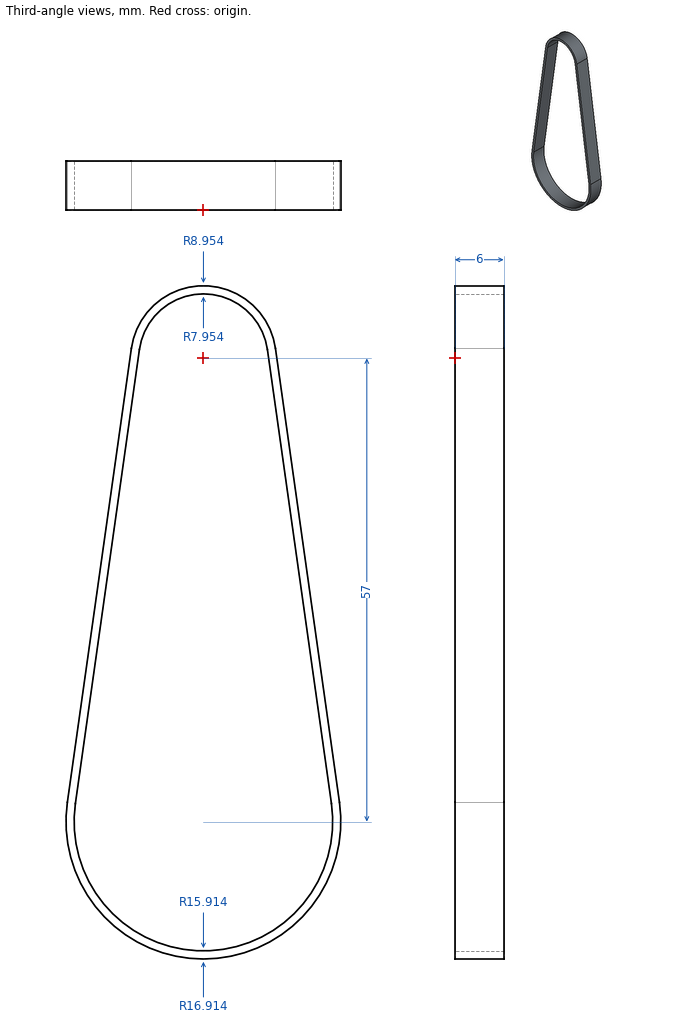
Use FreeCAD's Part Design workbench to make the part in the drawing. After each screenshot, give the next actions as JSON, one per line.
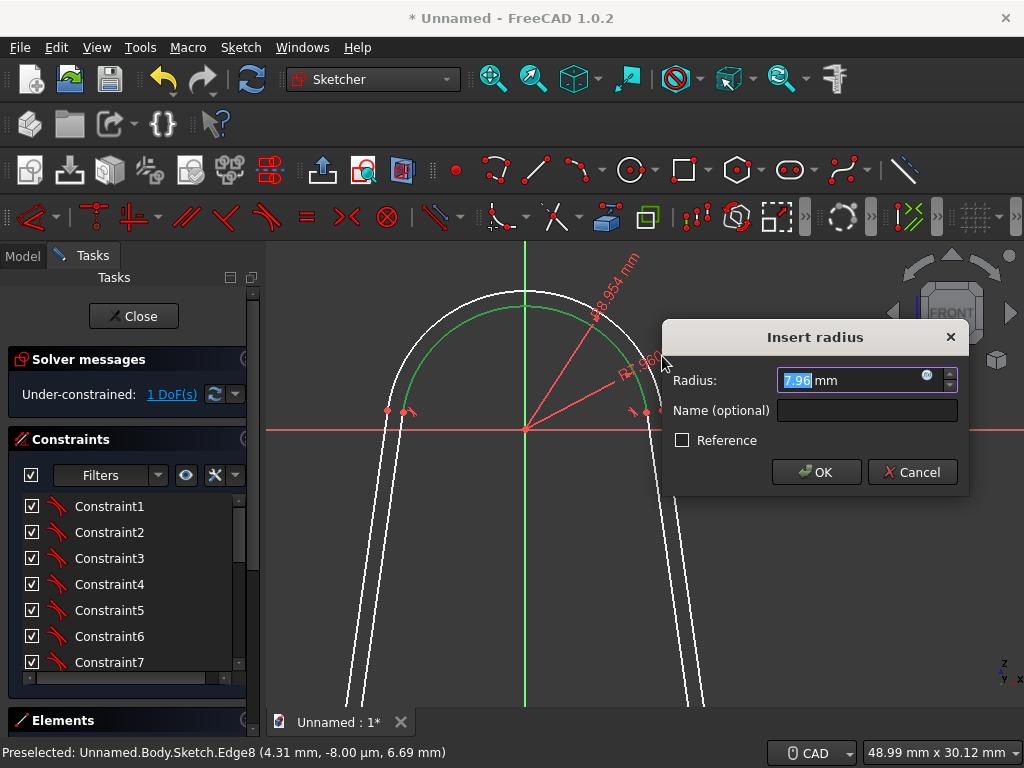
{"action": "type", "text": "7.954"}
{"action": "key", "text": "Return"}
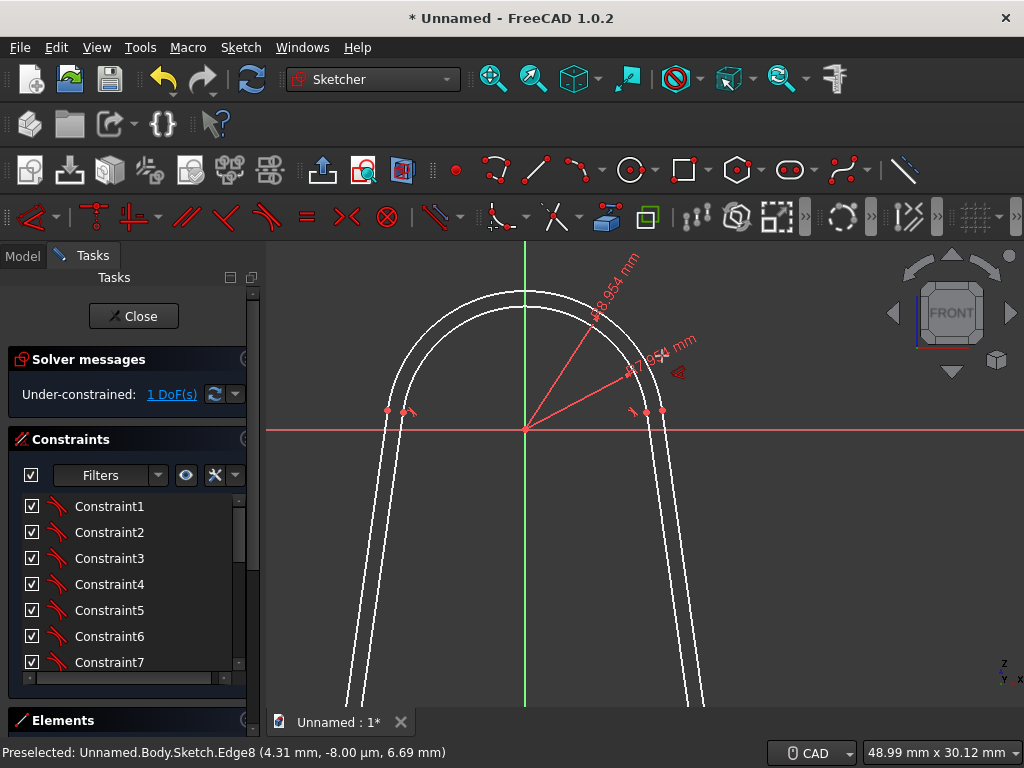
{"action": "scroll", "coordinate": [593, 324], "scroll_direction": "down", "scroll_amount": 7}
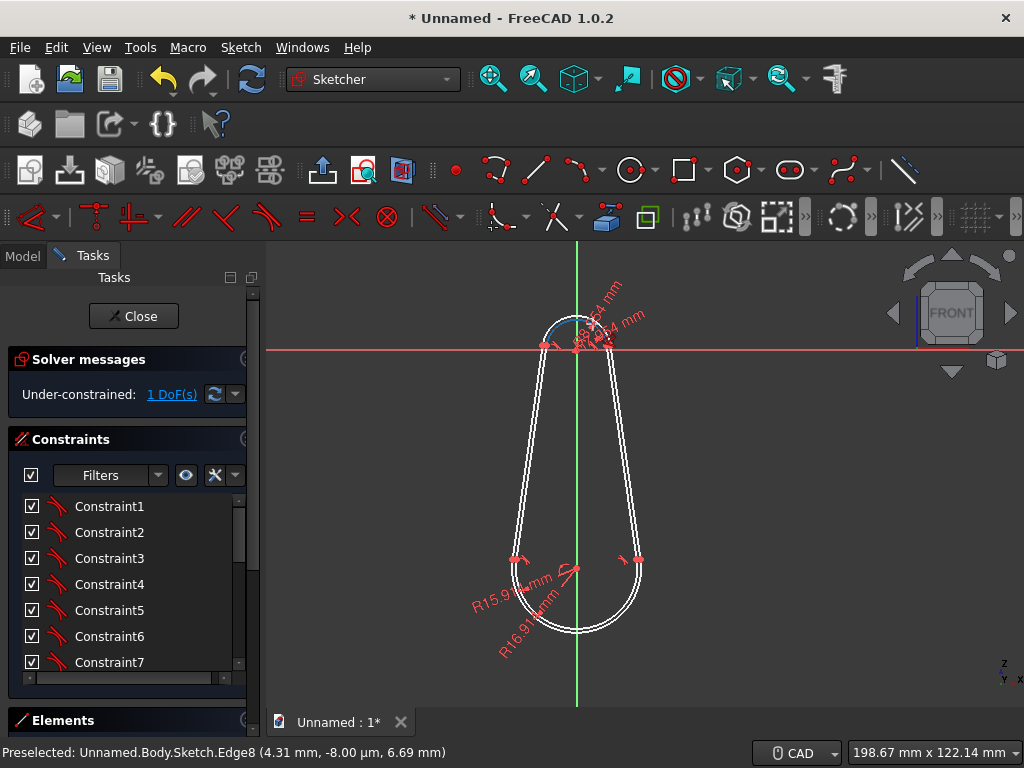
{"action": "left_click", "coordinate": [577, 568]}
{"action": "left_click", "coordinate": [611, 509]}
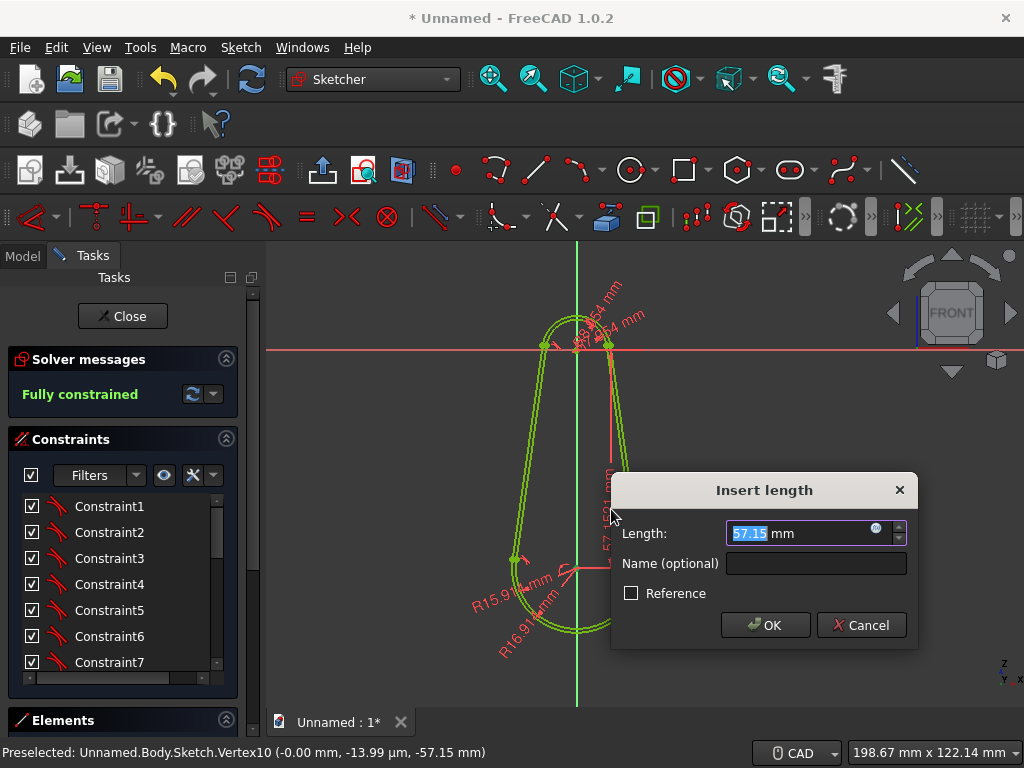
{"action": "type", "text": "57"}
{"action": "key", "text": "Return"}
{"action": "key", "text": "Escape"}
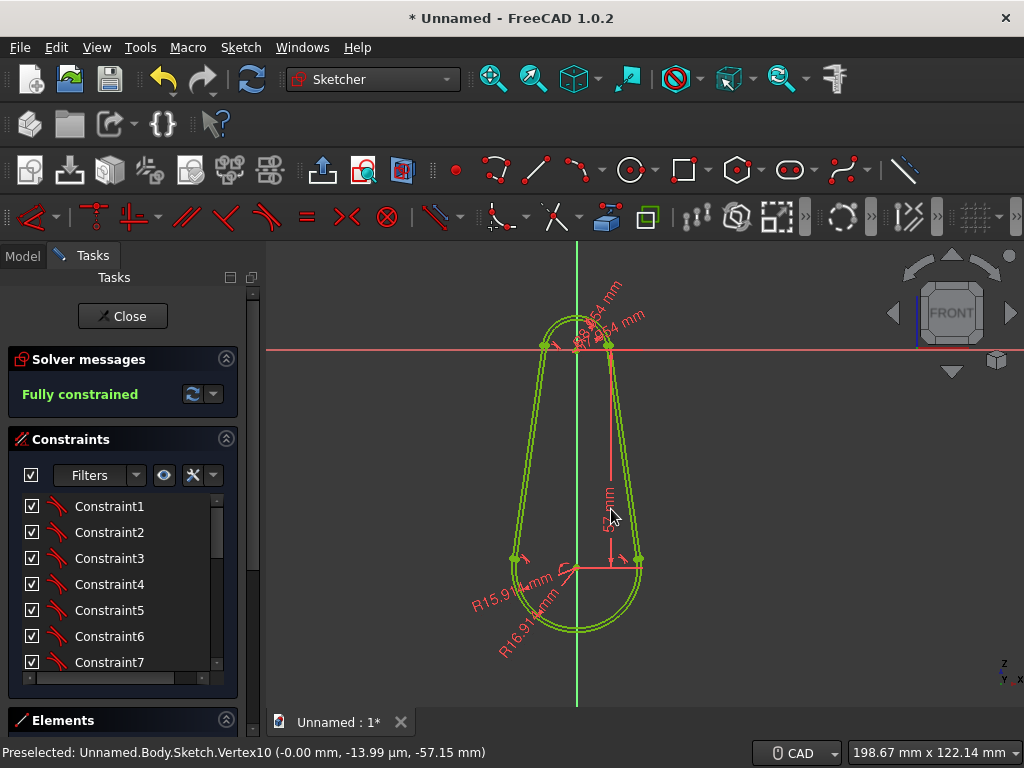
{"action": "left_click", "coordinate": [123, 316]}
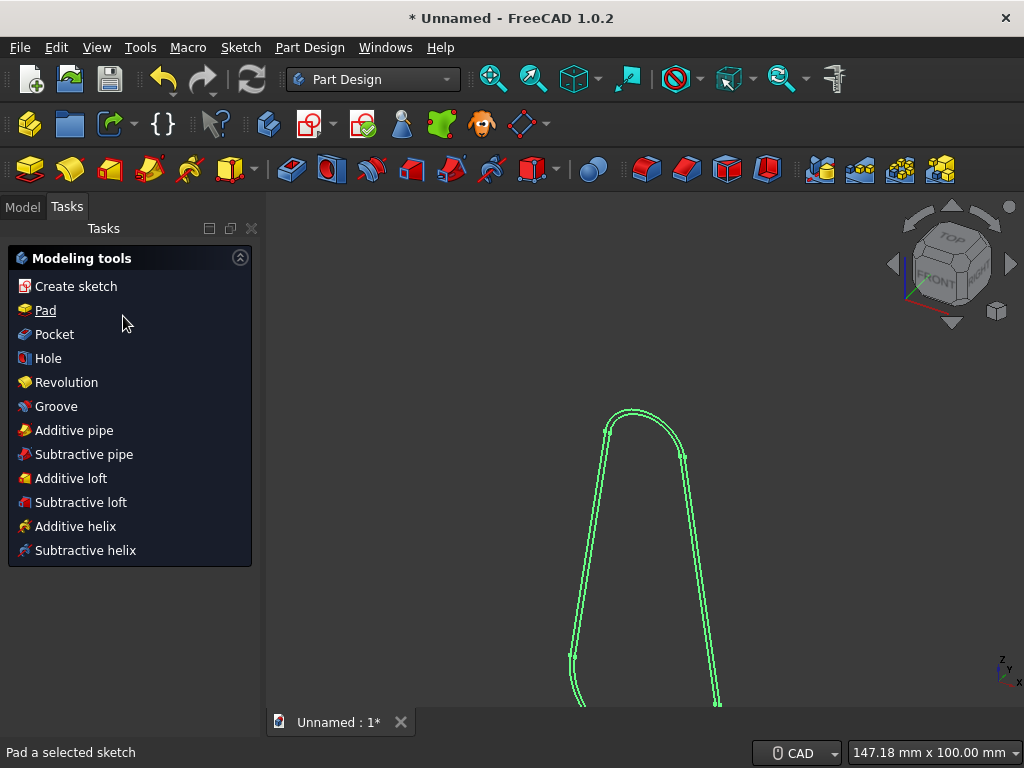
{"action": "left_click", "coordinate": [30, 170]}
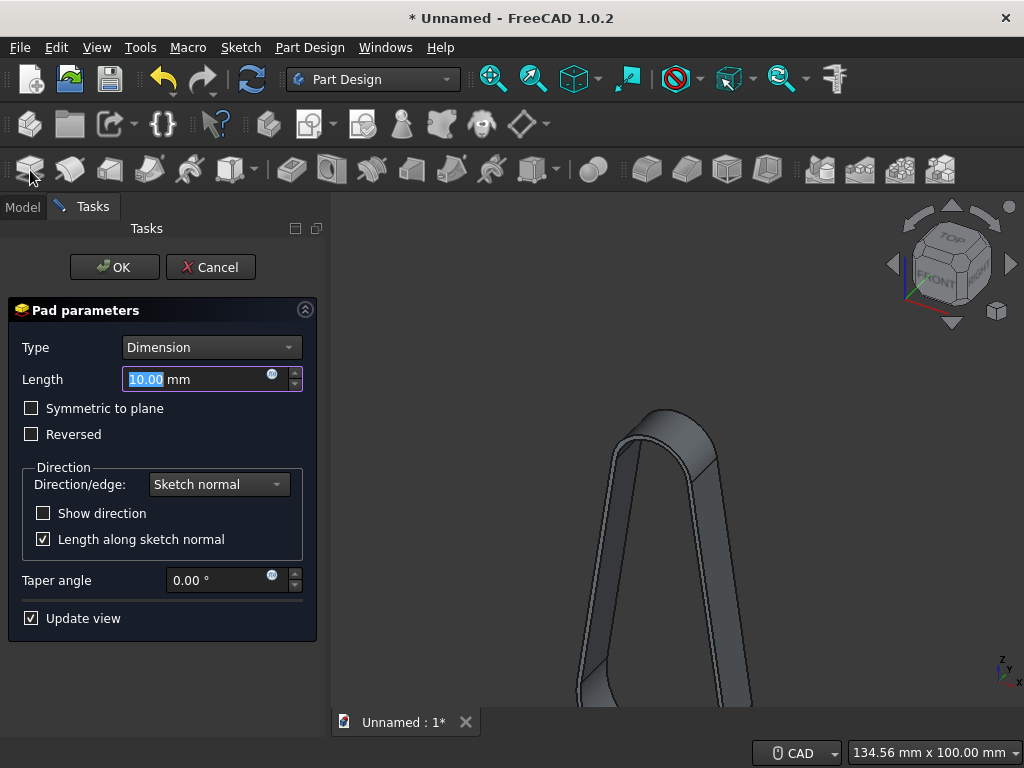
{"action": "type", "text": "6"}
{"action": "key", "text": "Tab"}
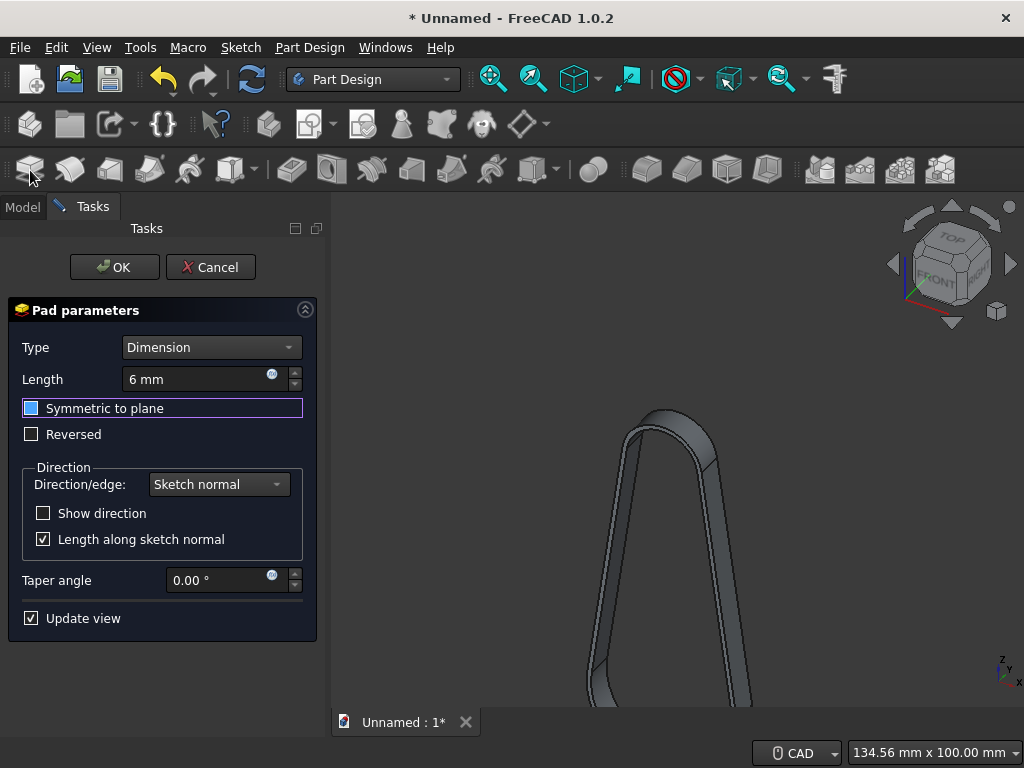
{"action": "left_click", "coordinate": [30, 434]}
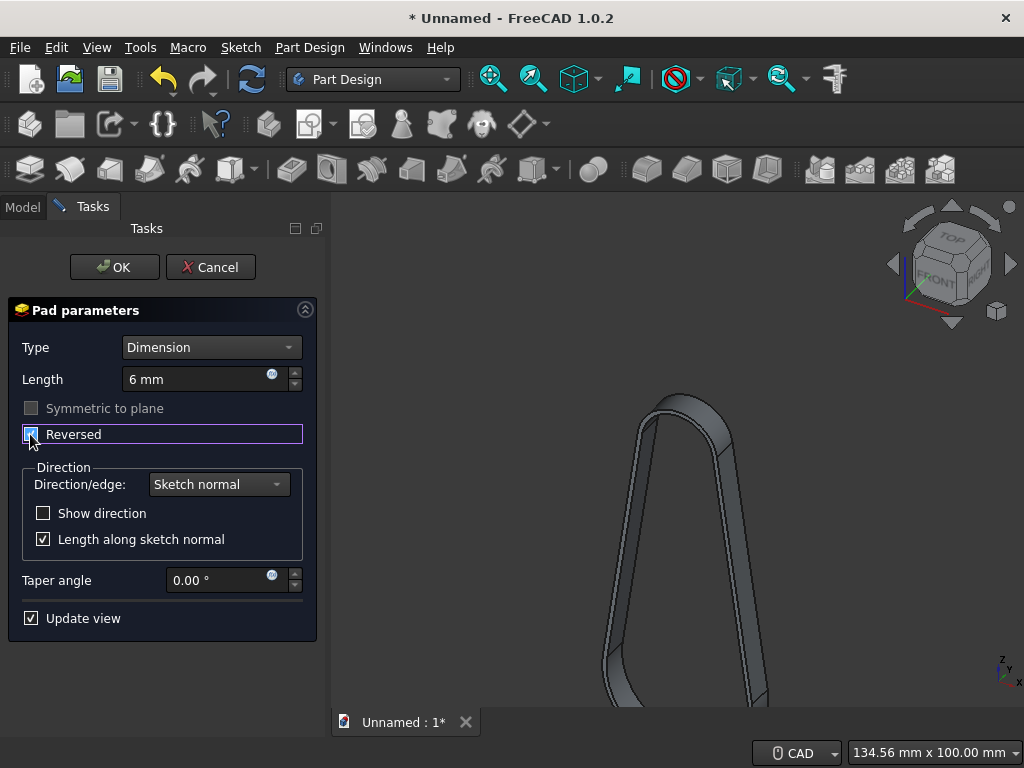
{"action": "left_click", "coordinate": [115, 267]}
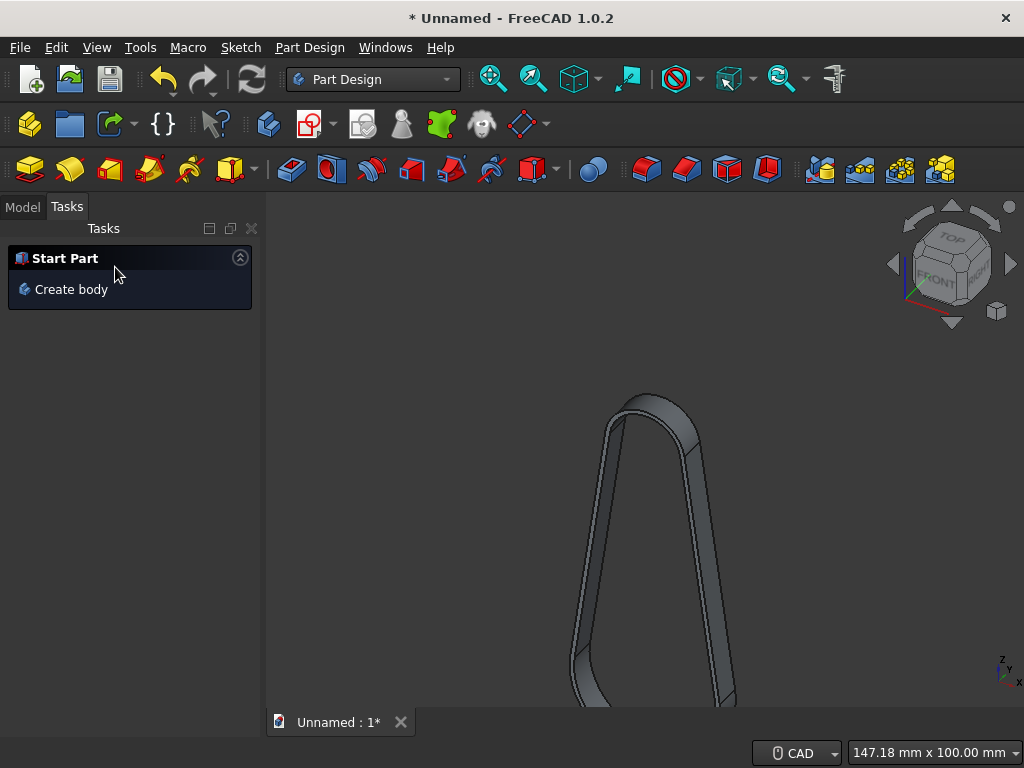
{"action": "key", "text": "0"}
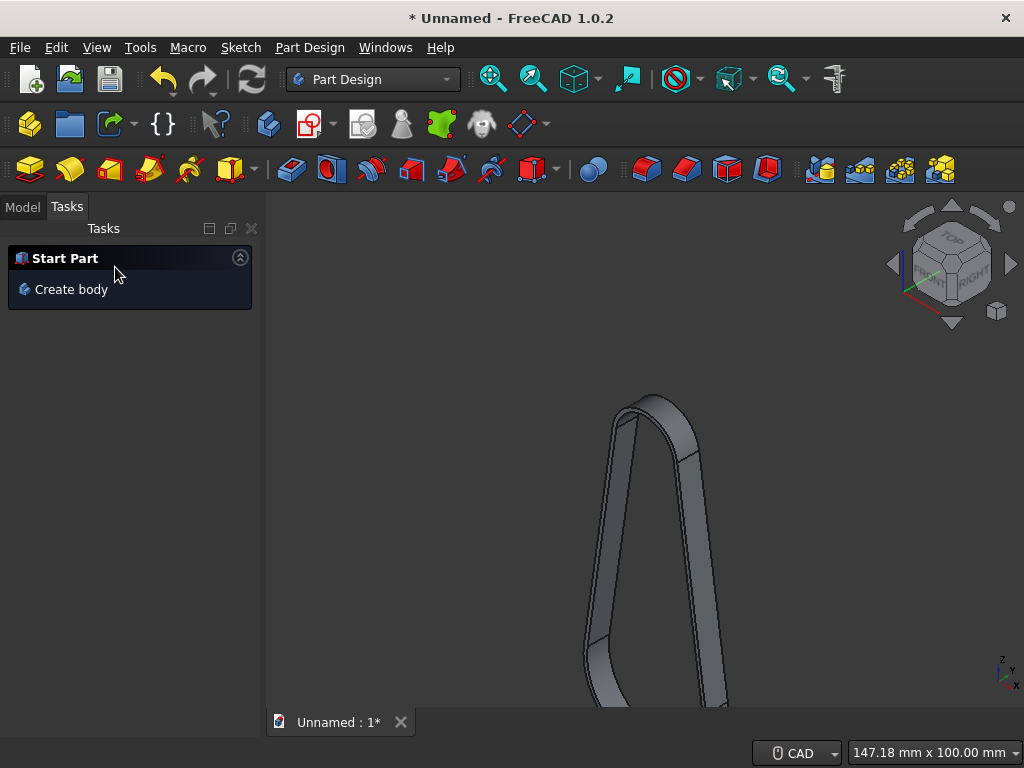
{"action": "left_click", "coordinate": [494, 80]}